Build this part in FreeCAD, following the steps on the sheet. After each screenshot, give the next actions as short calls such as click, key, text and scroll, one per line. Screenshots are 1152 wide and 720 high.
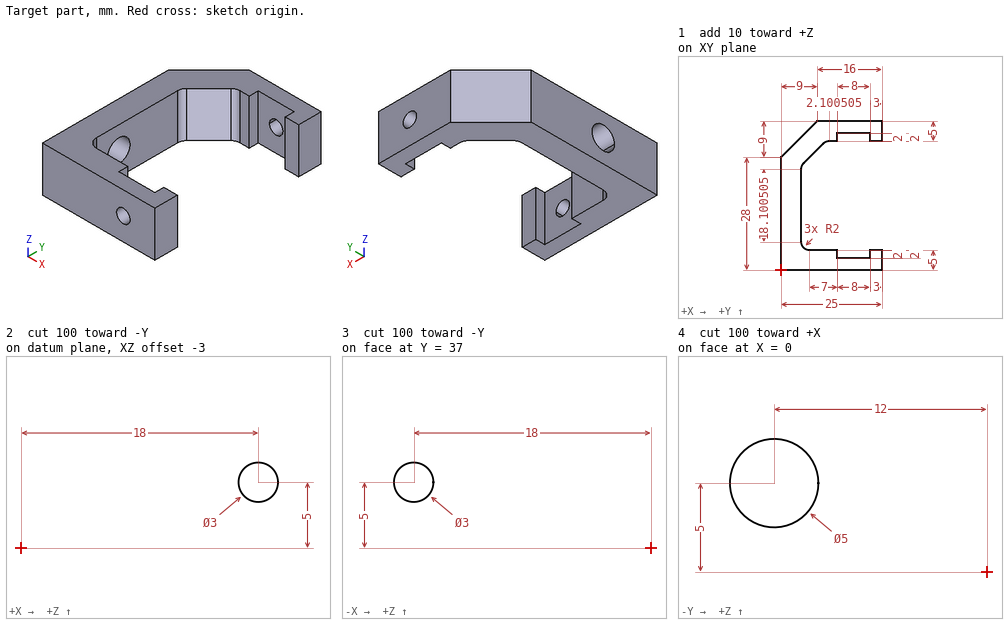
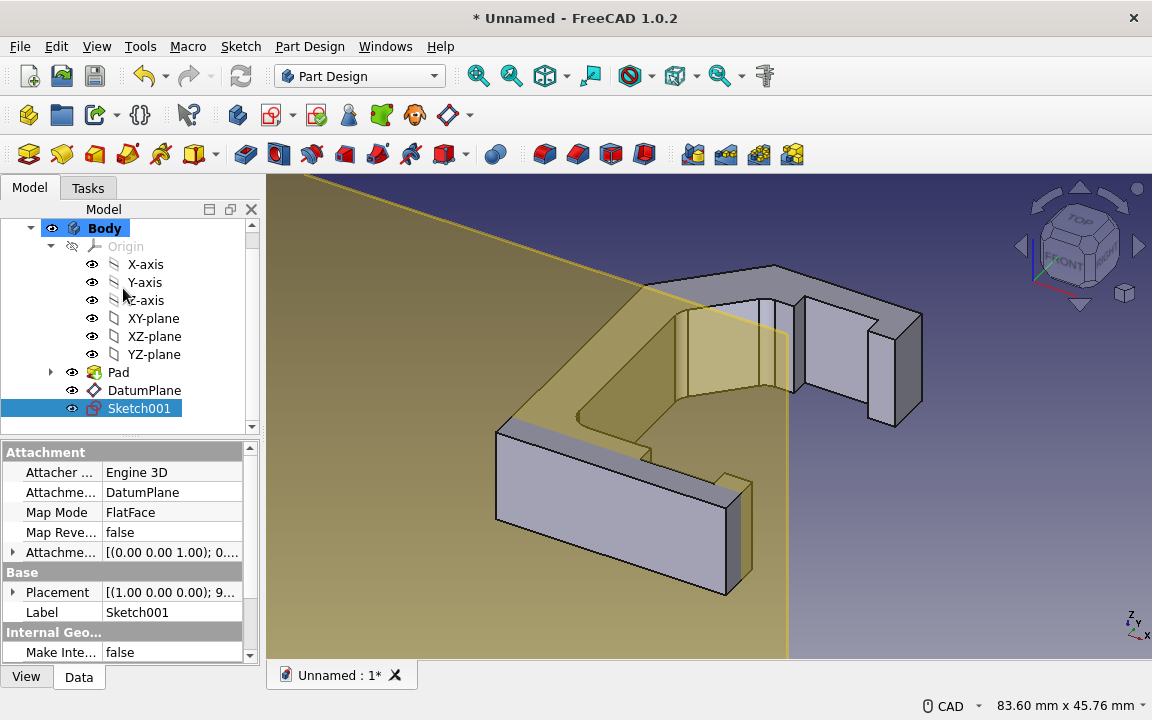
click(246, 154)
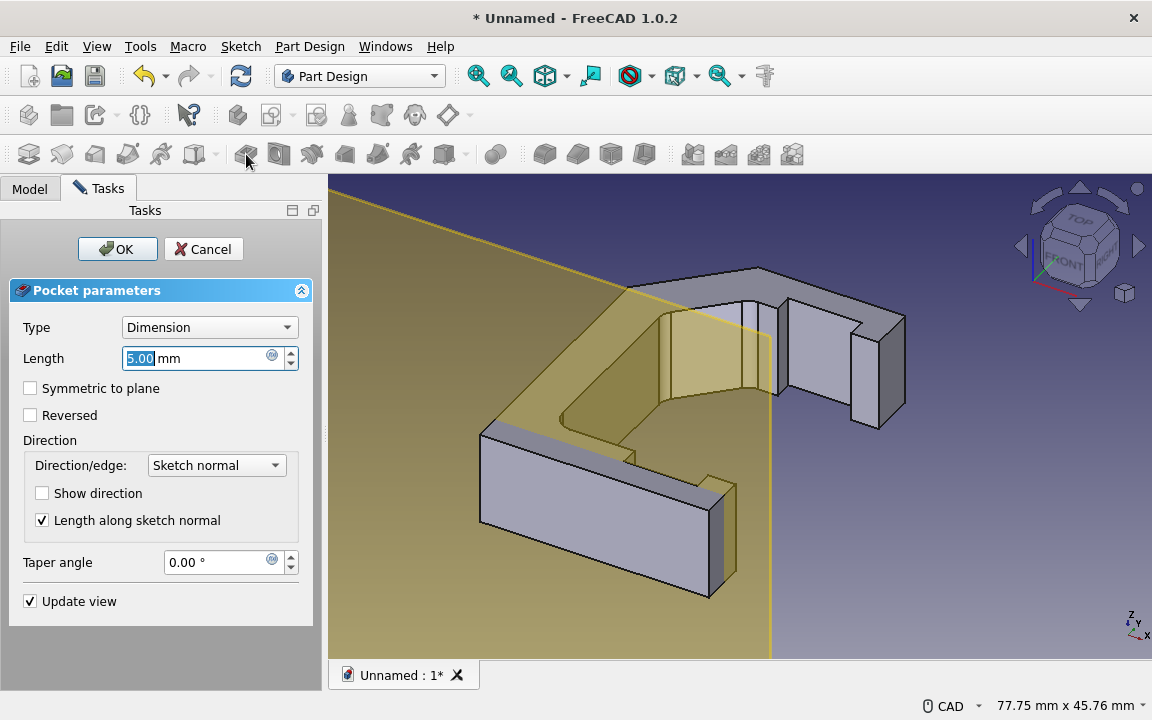
text(100)
key(Tab)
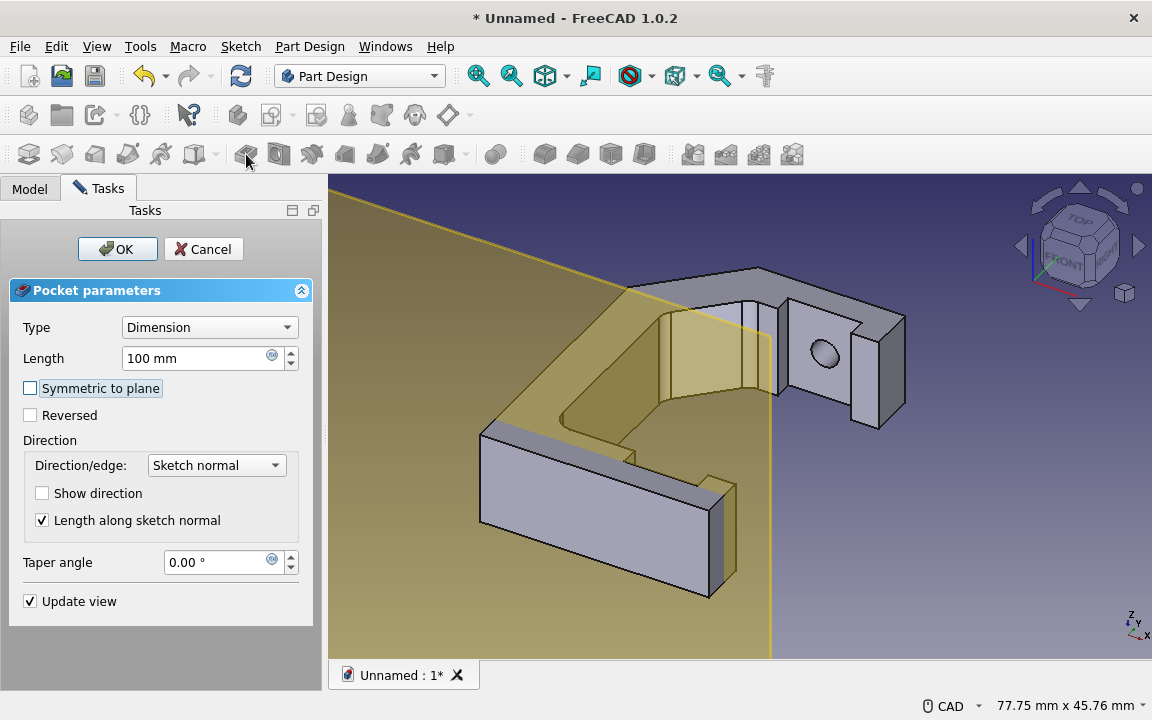
click(31, 415)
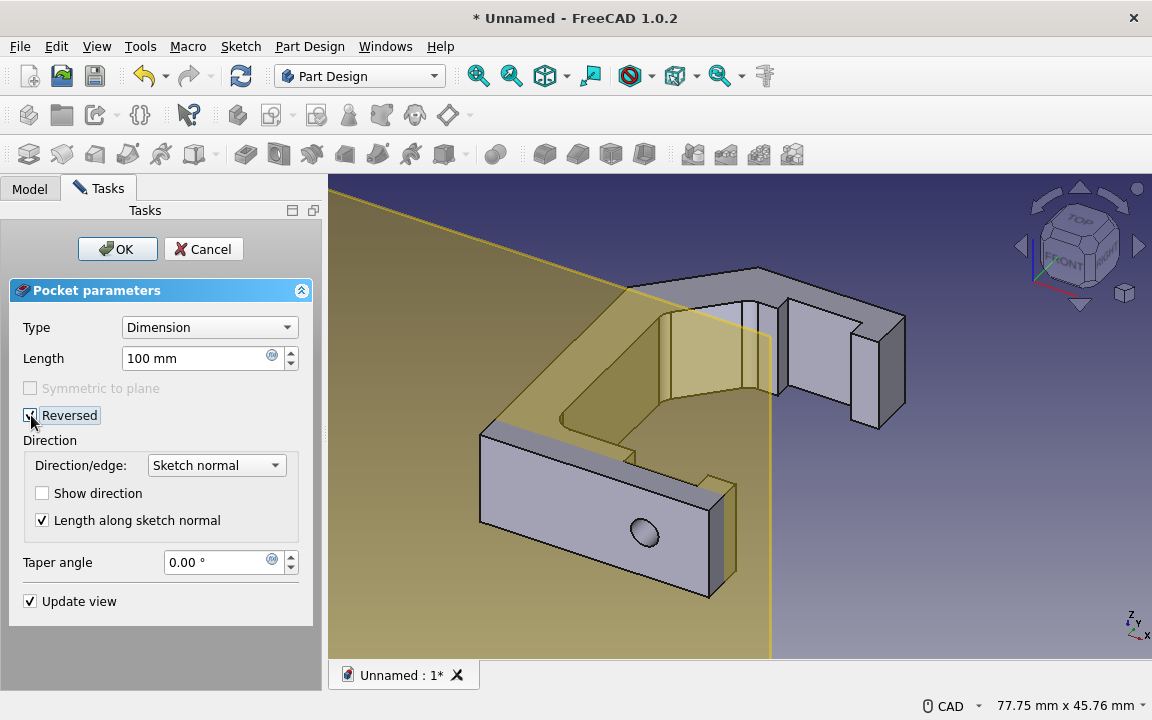
click(118, 249)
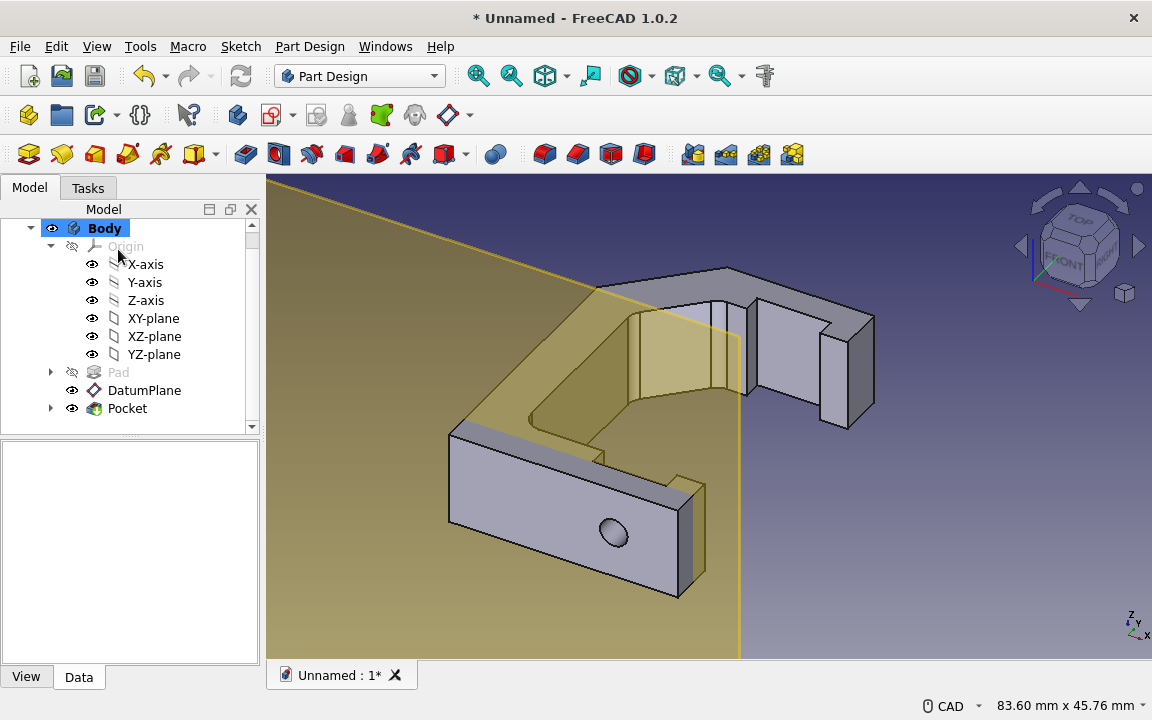
click(117, 390)
key(space)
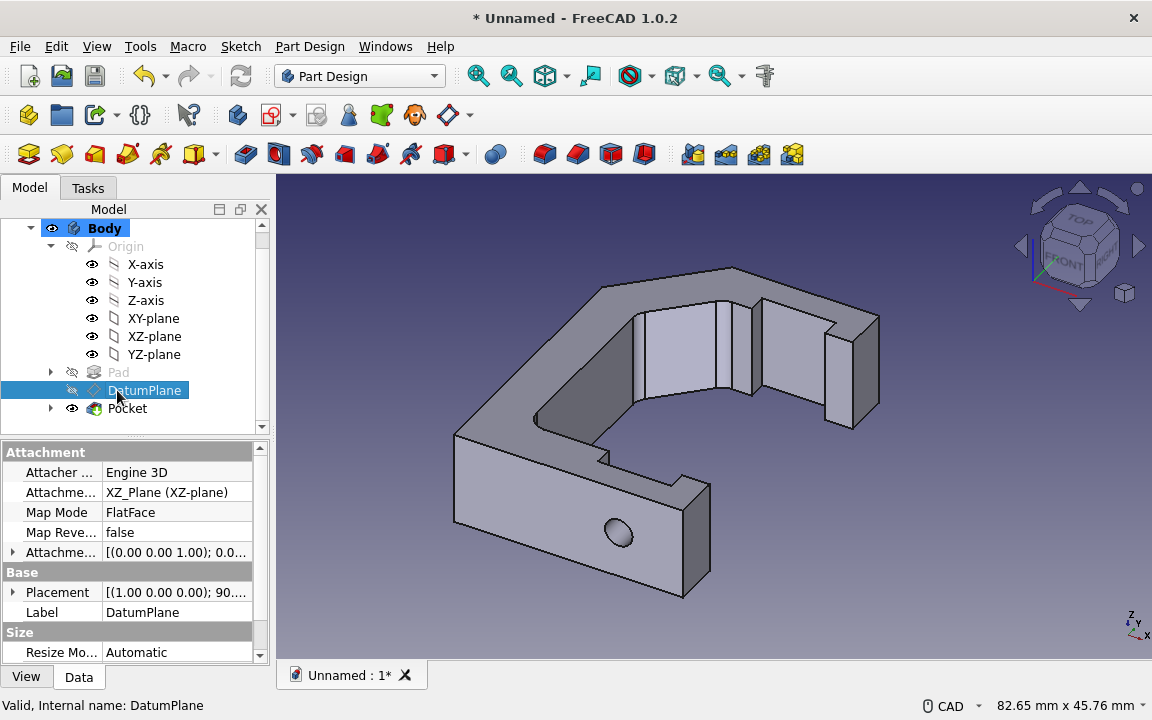
key(4)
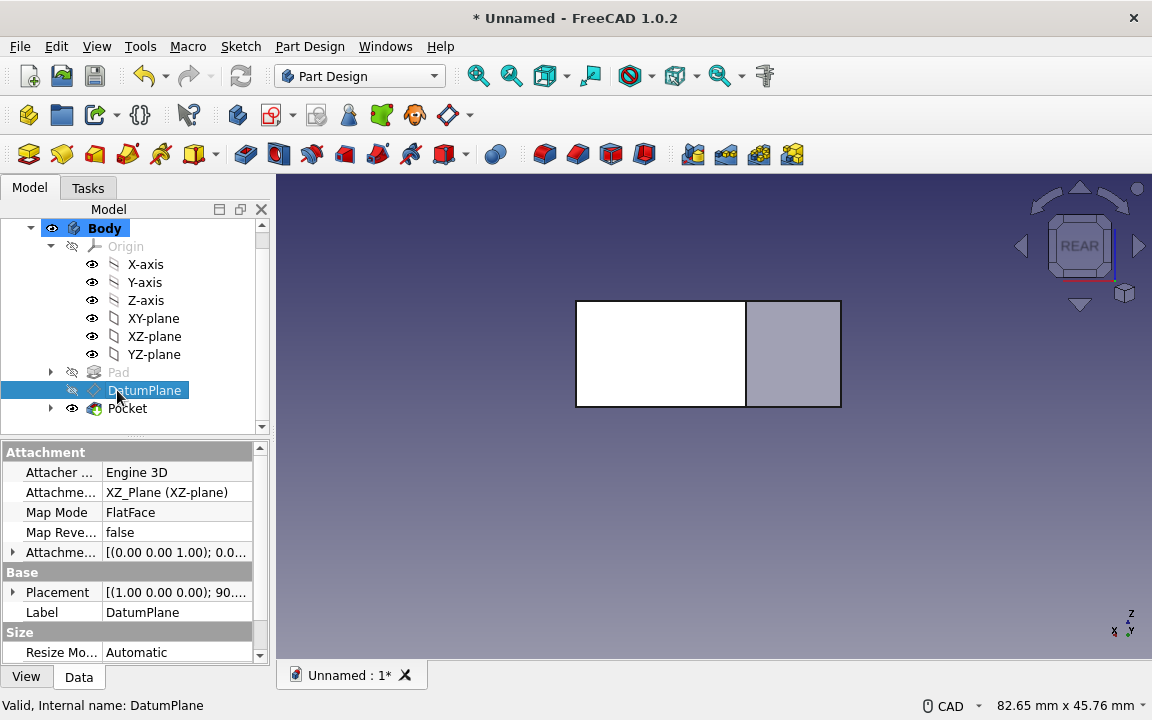
key(v)
key(f)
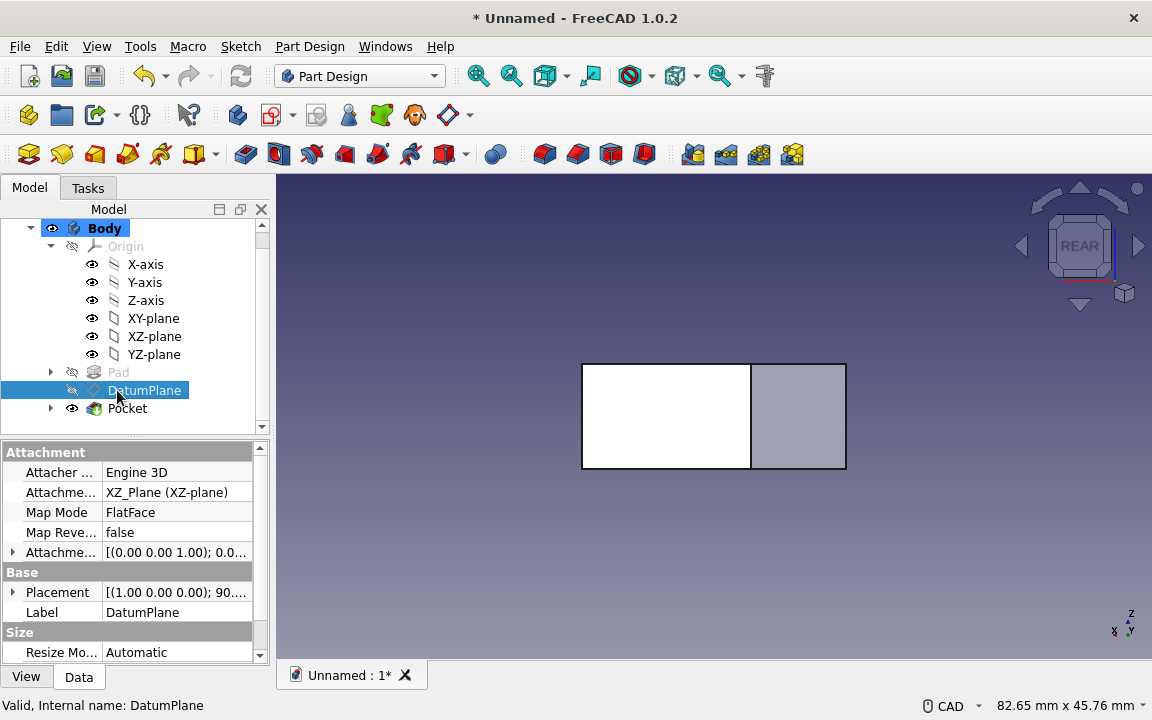
click(642, 416)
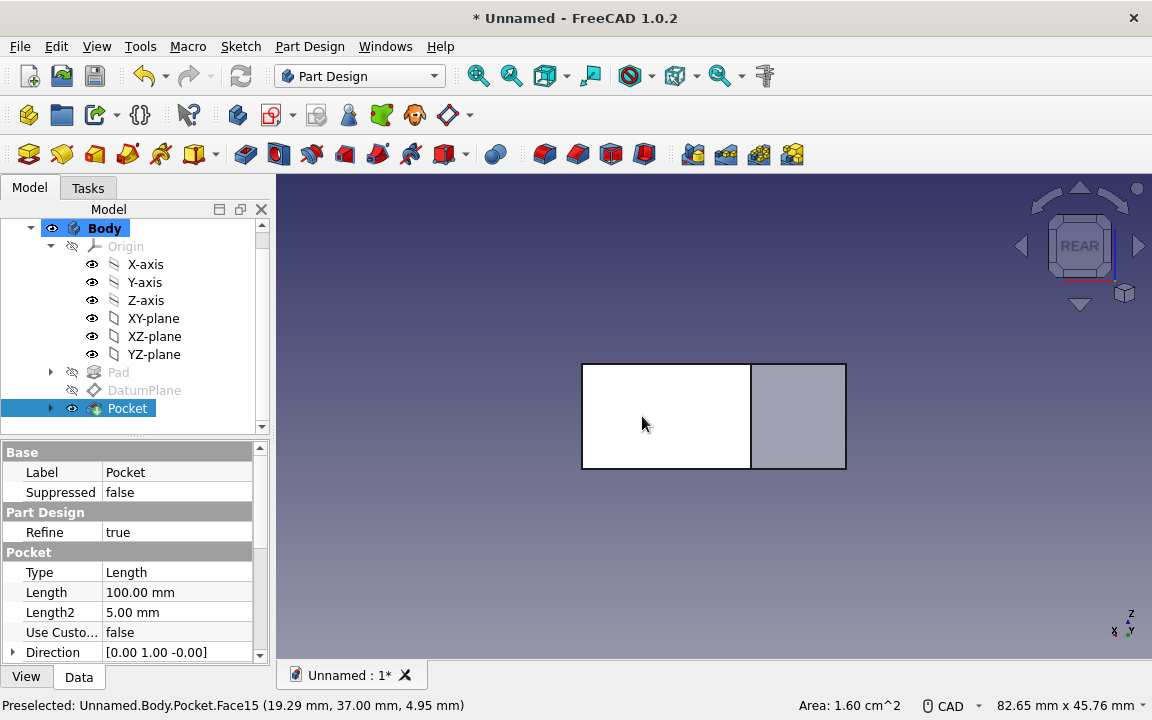
click(270, 116)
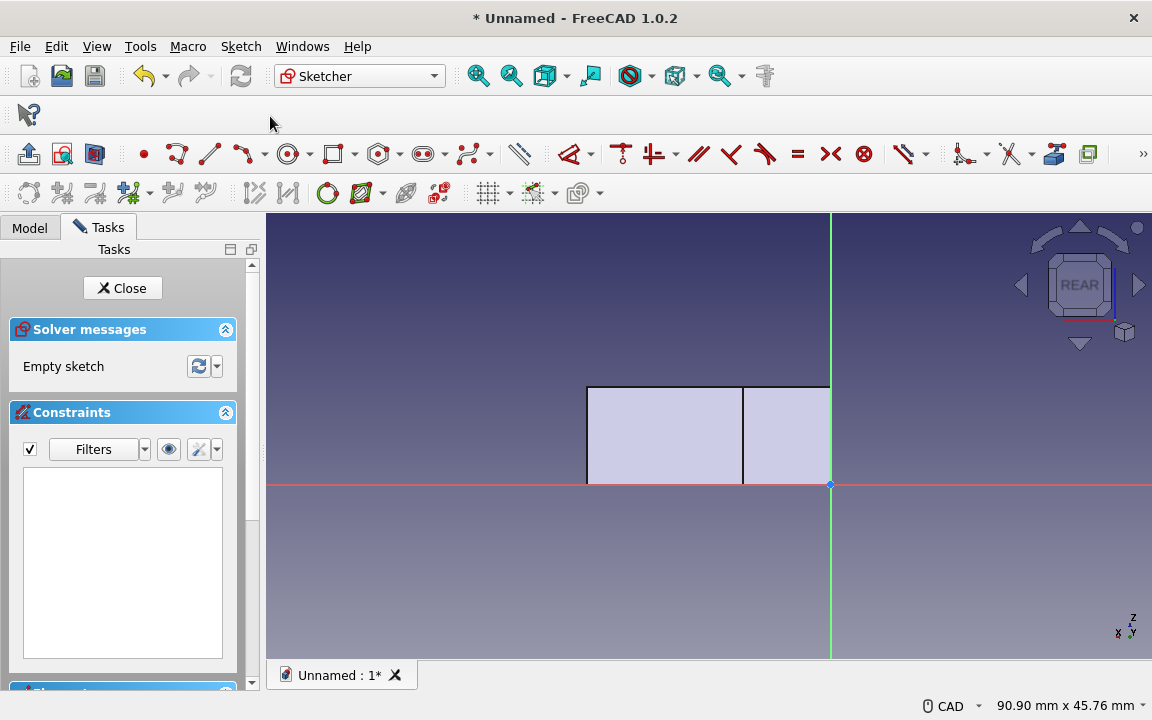
scroll(657, 436, up, 11)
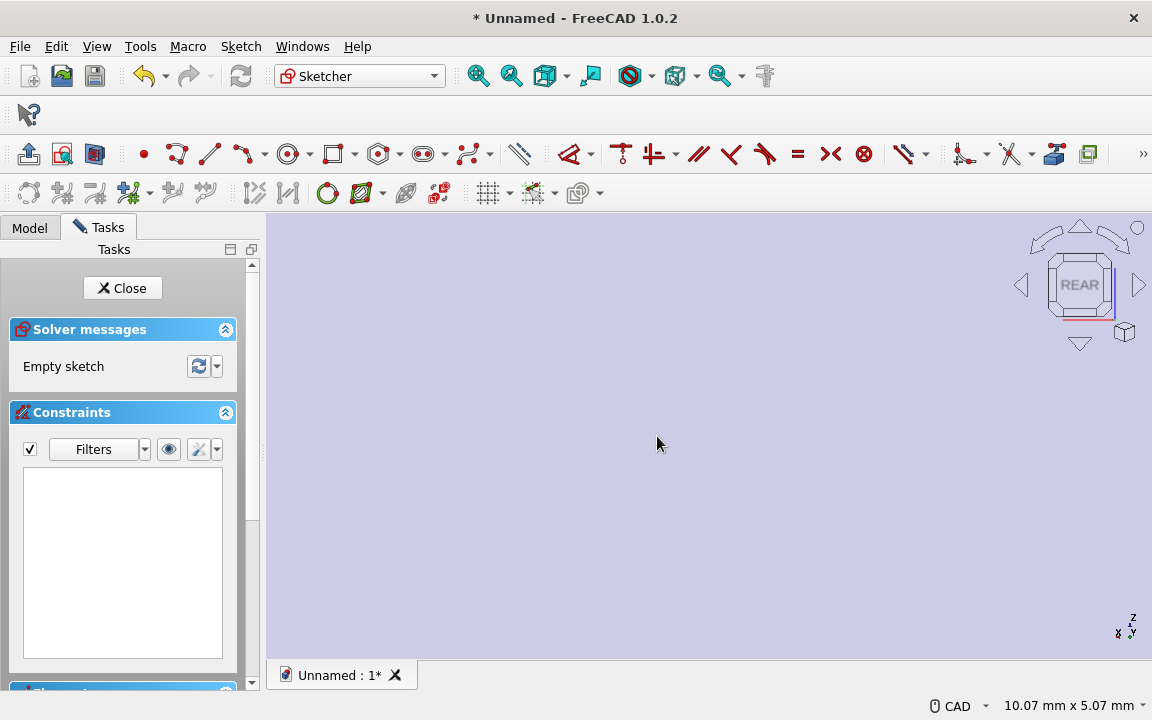
key(g)
key(c)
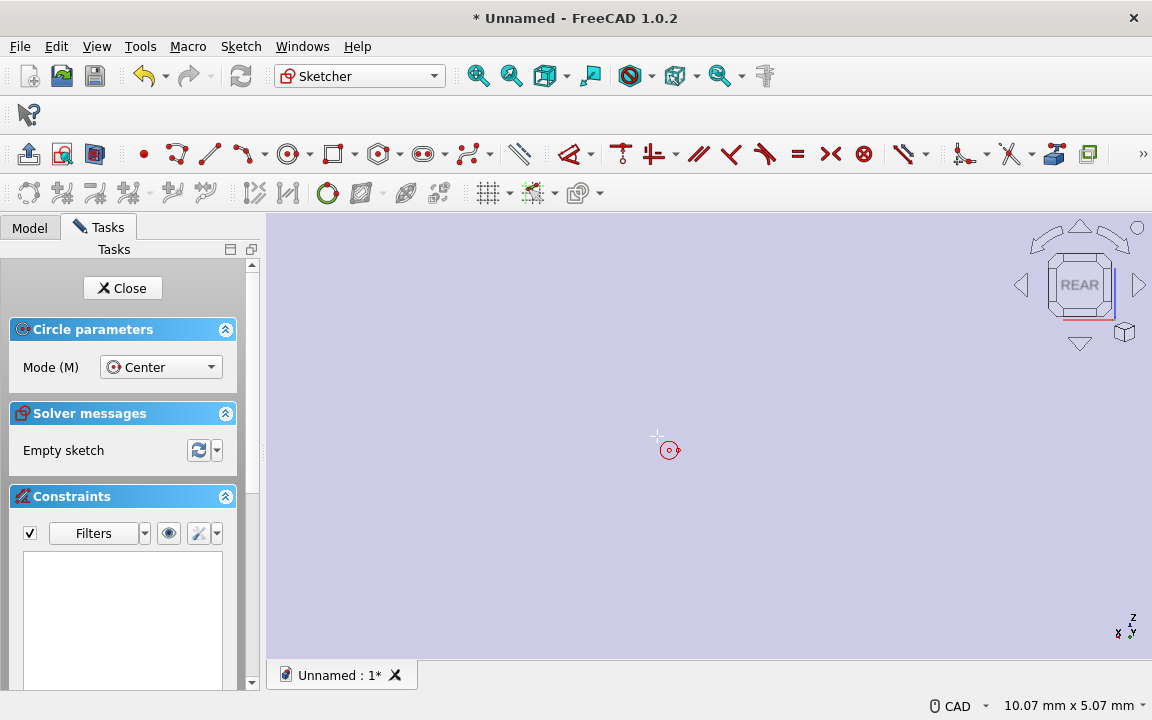
click(639, 432)
click(732, 339)
key(Escape)